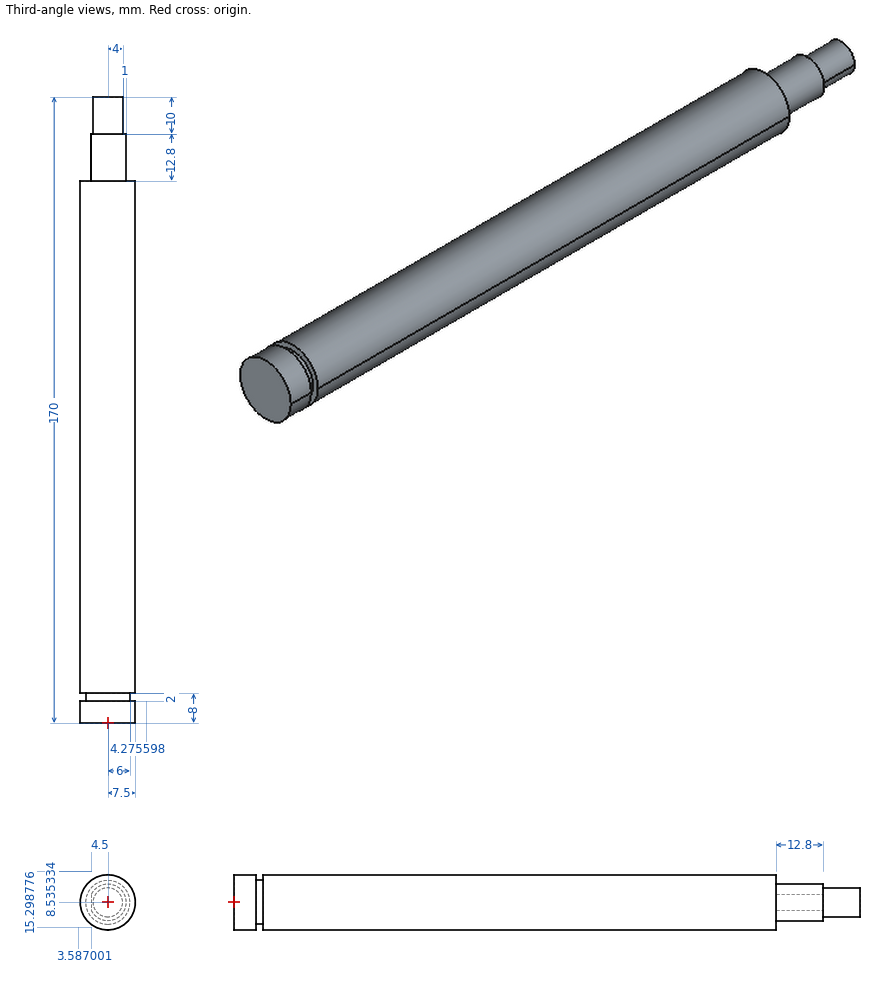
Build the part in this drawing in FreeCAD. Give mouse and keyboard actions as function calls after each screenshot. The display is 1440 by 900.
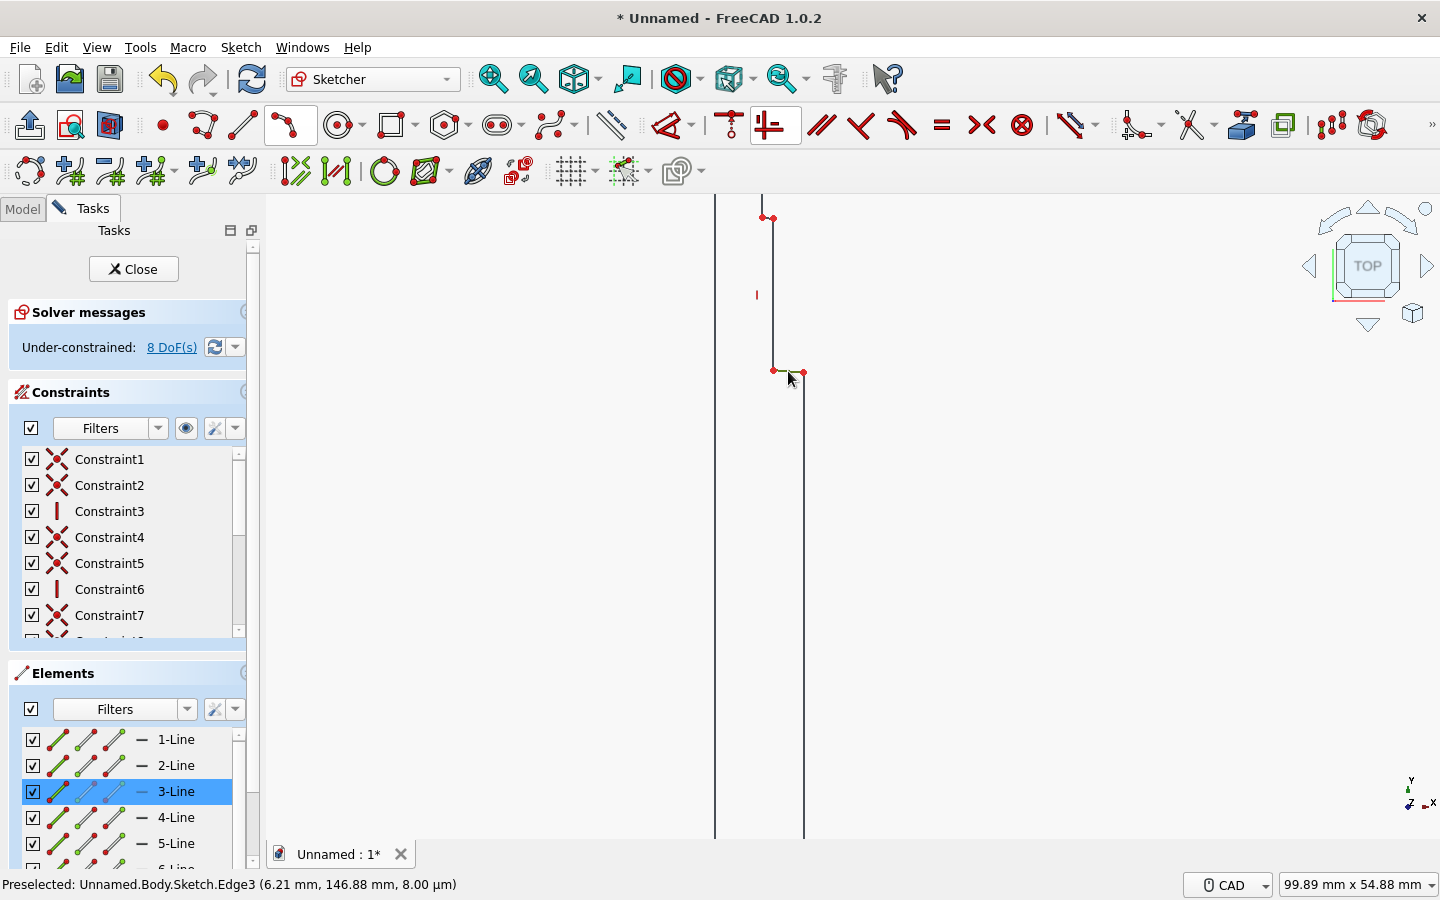
click(796, 126)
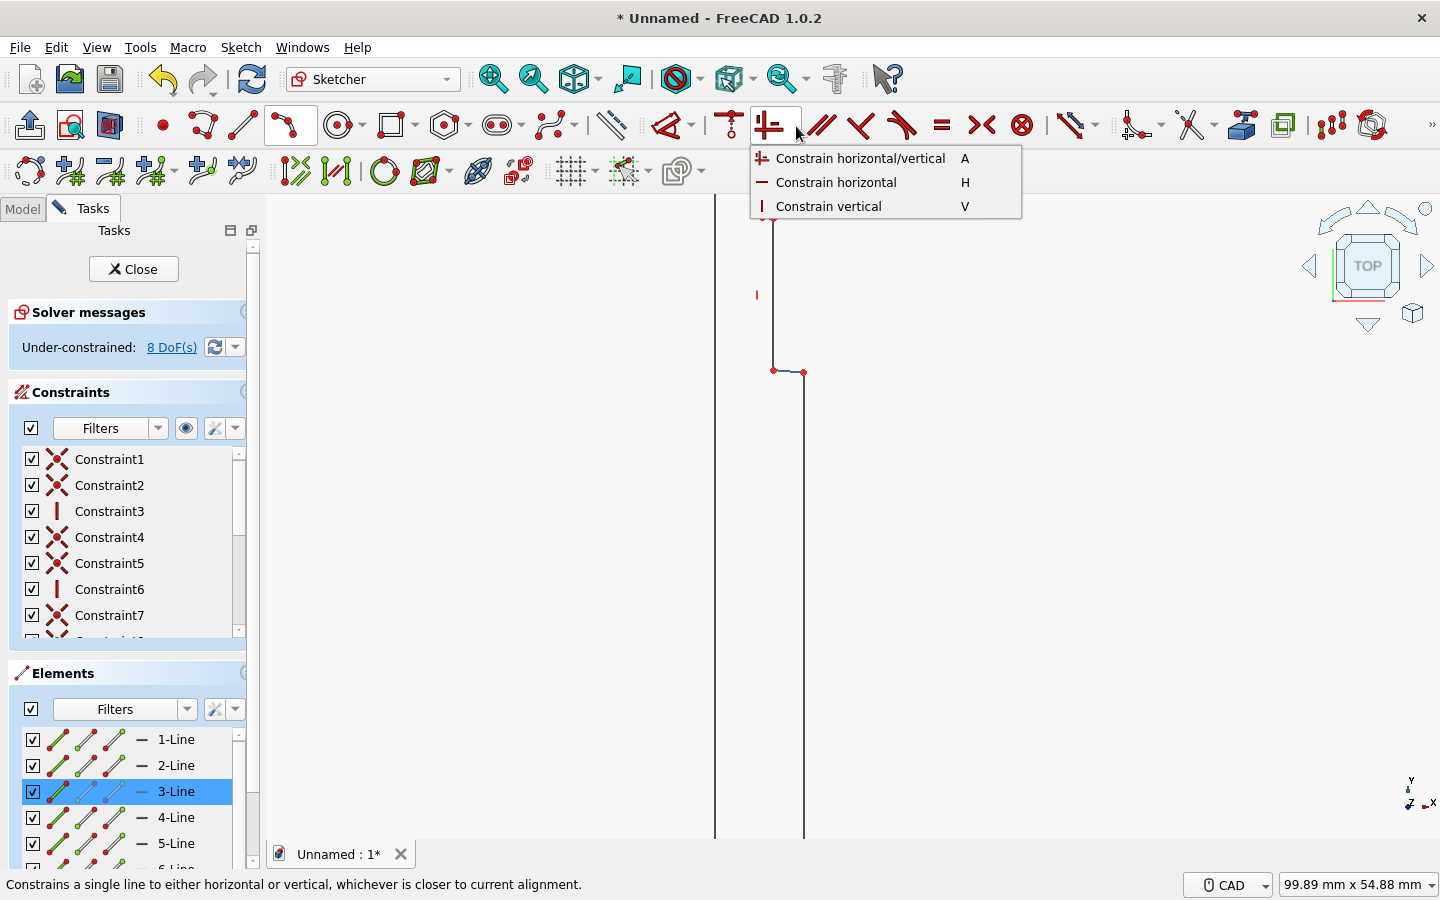
click(886, 182)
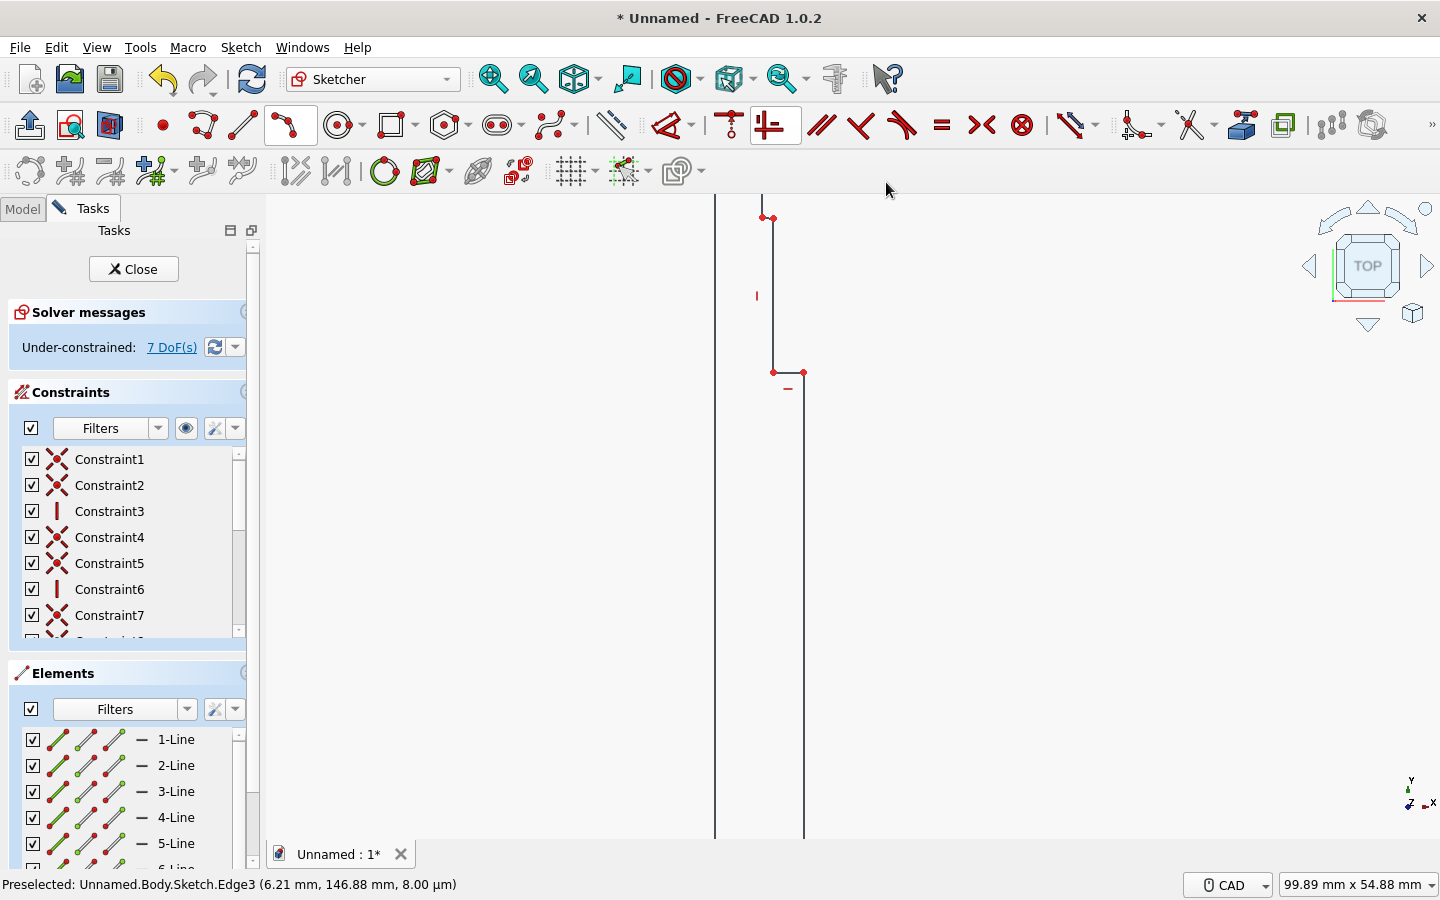
scroll(791, 369, down, 8)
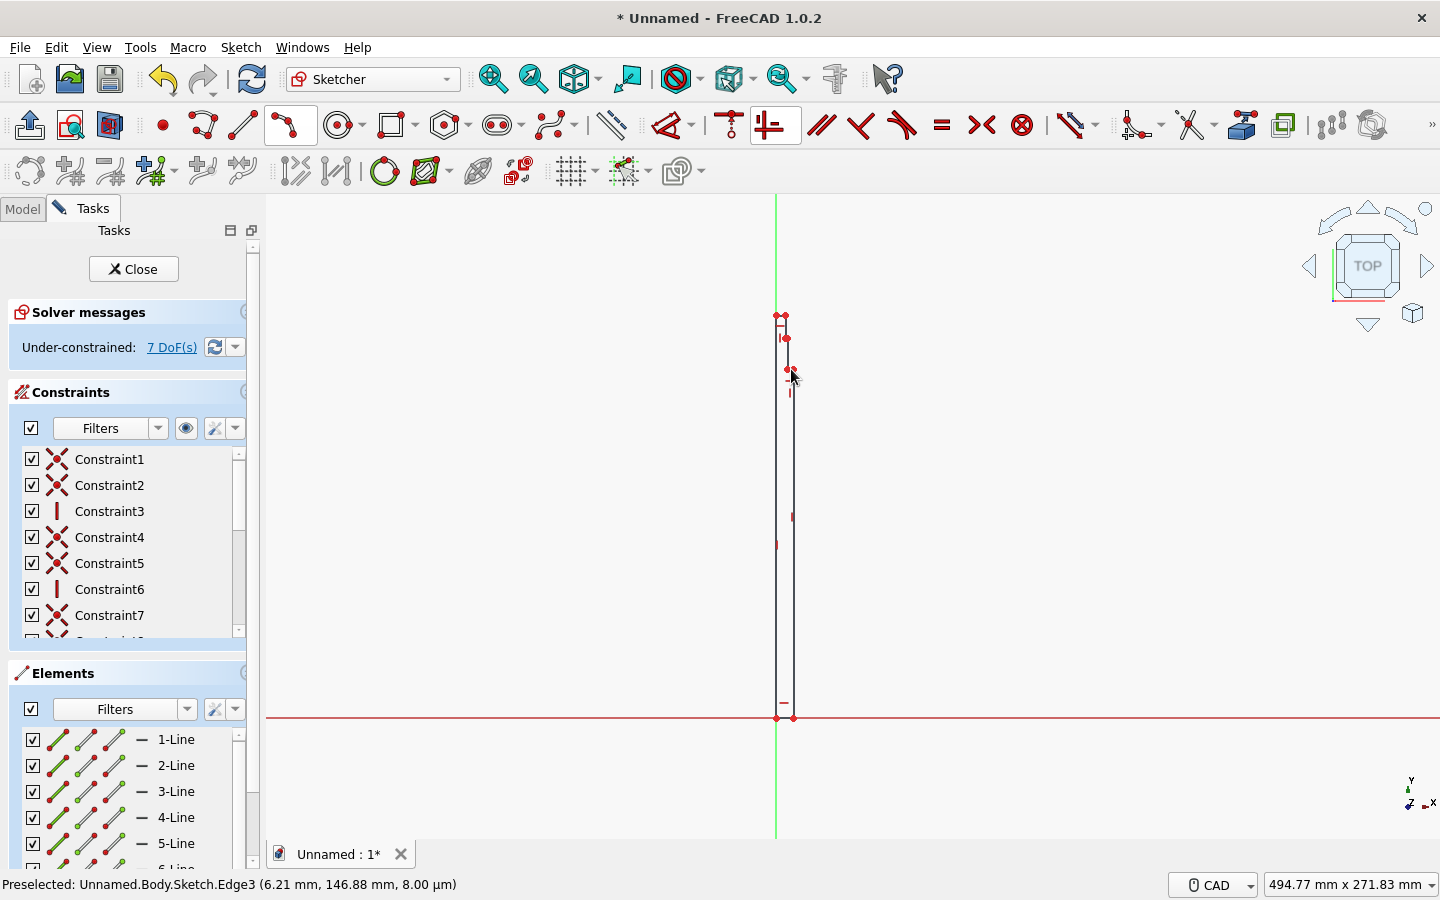
scroll(787, 339, up, 13)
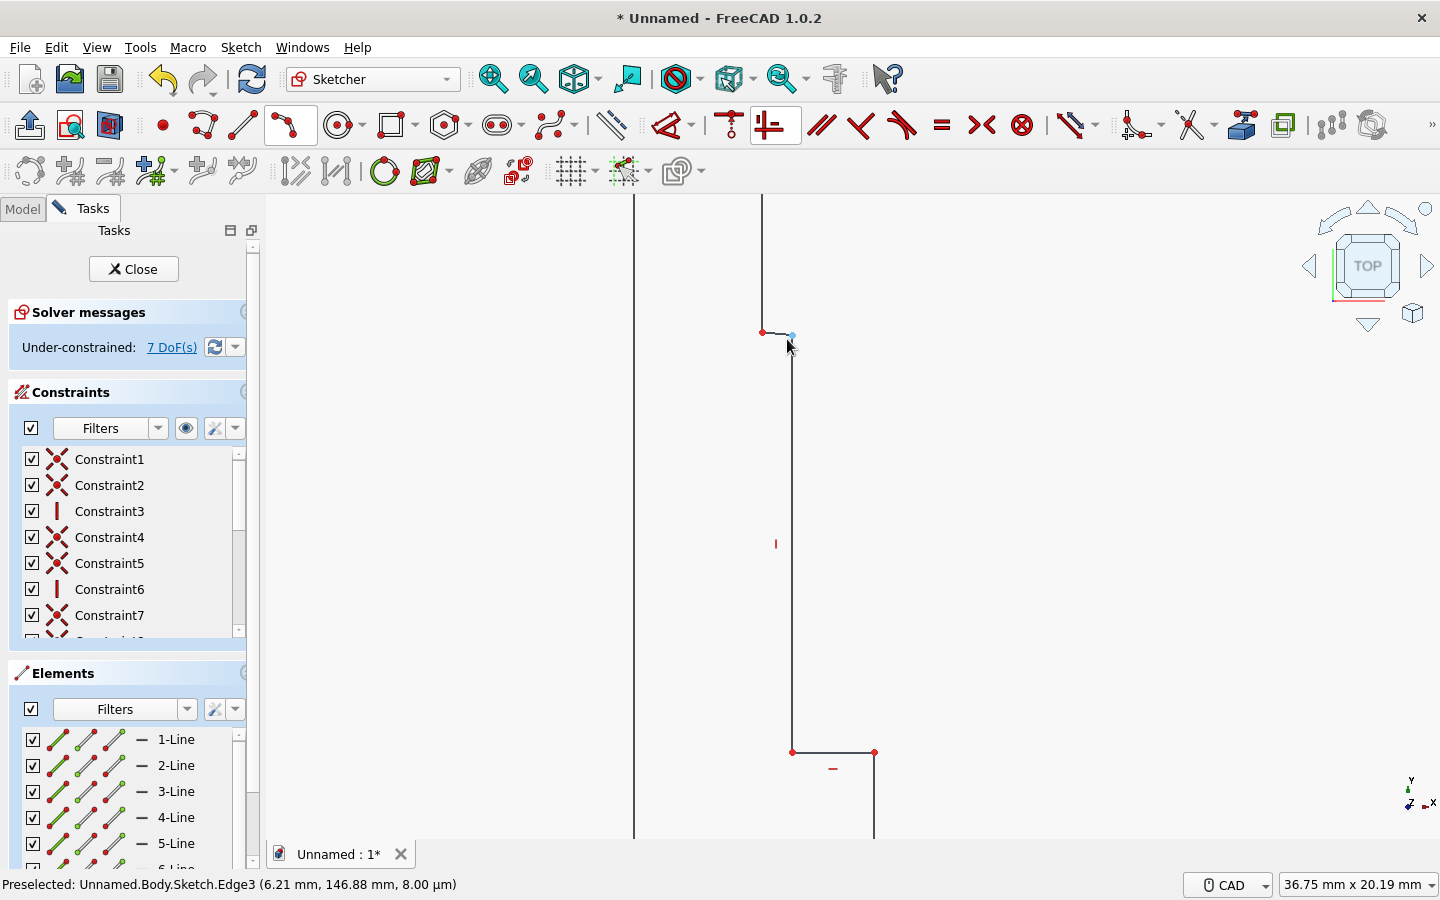
click(777, 334)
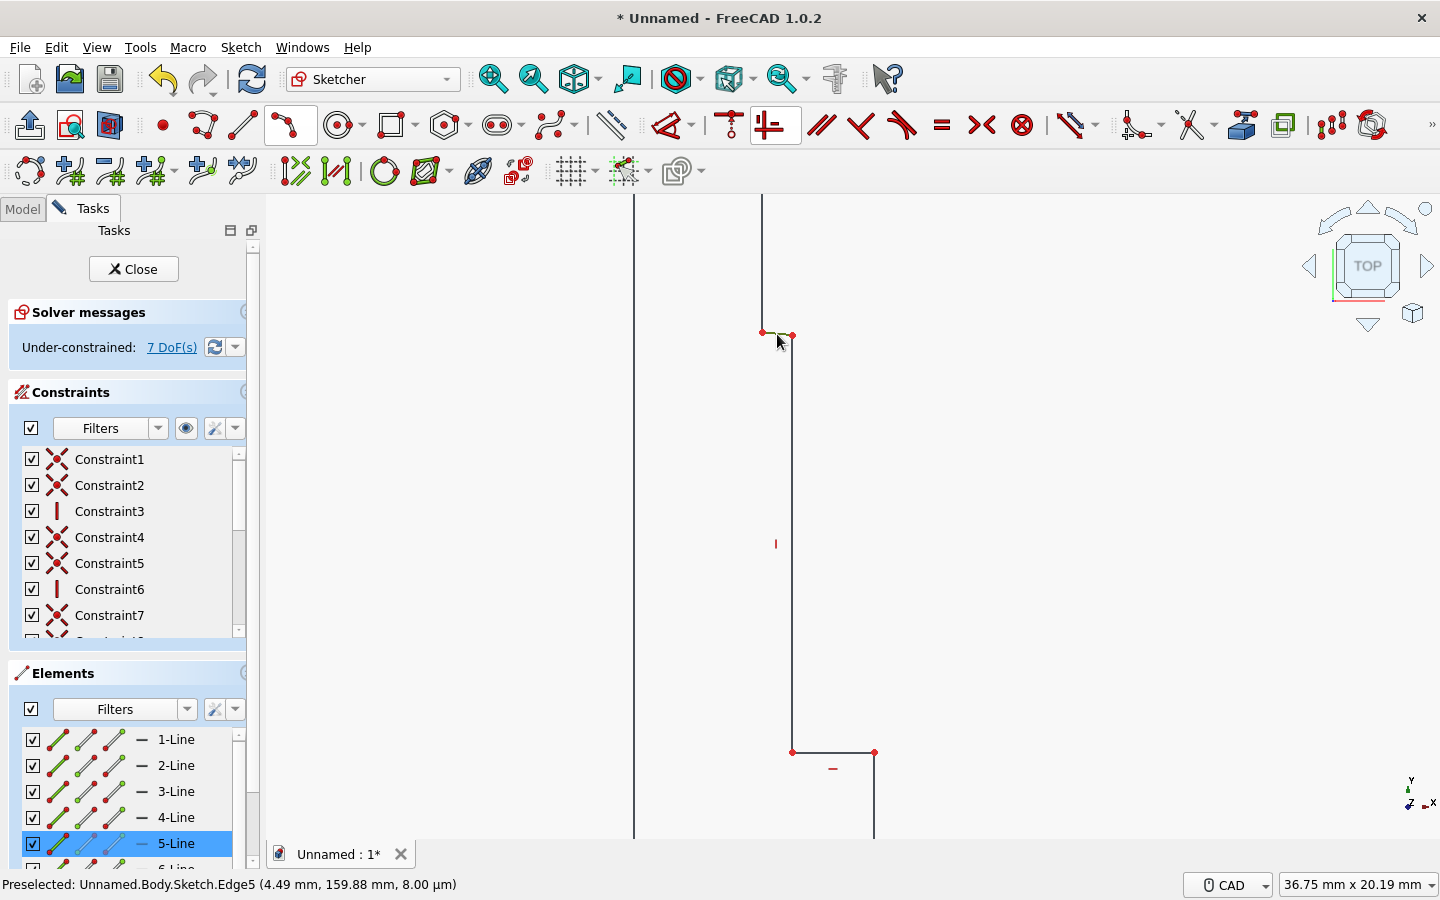
key(h)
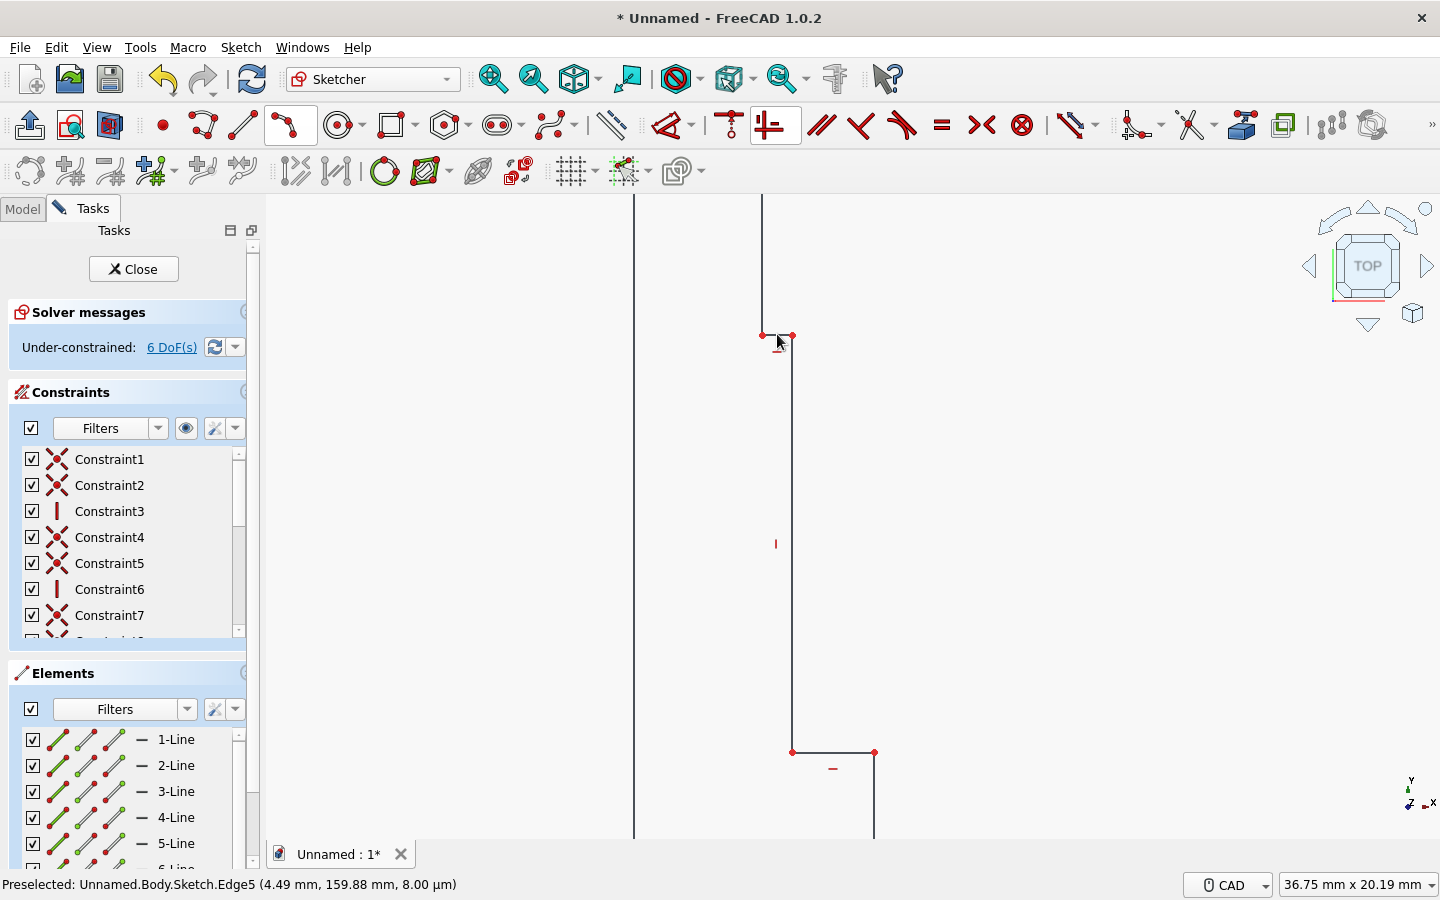
click(666, 126)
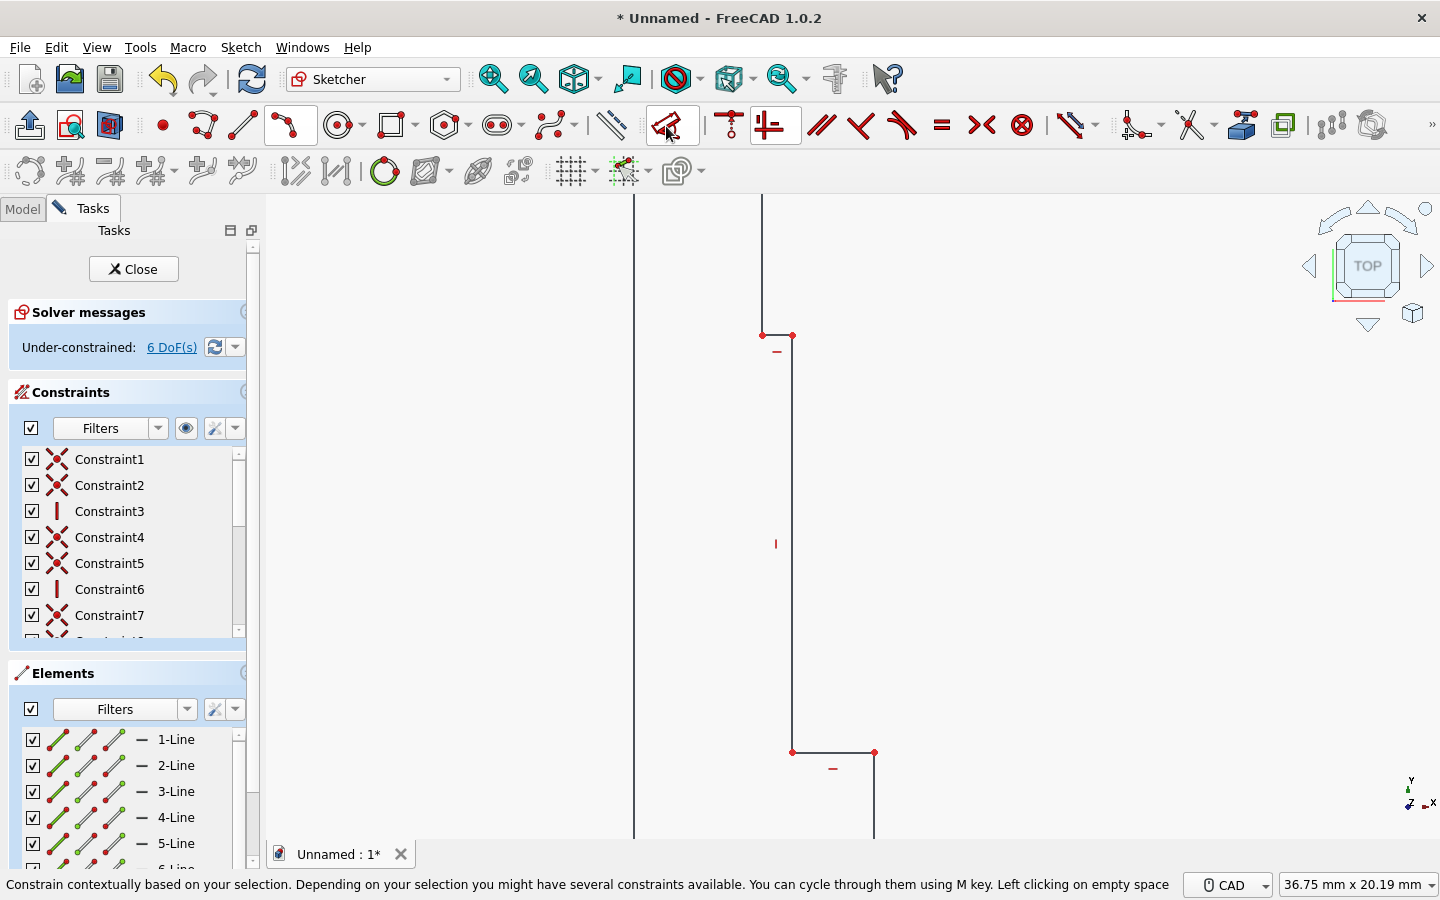
scroll(783, 335, up, 2)